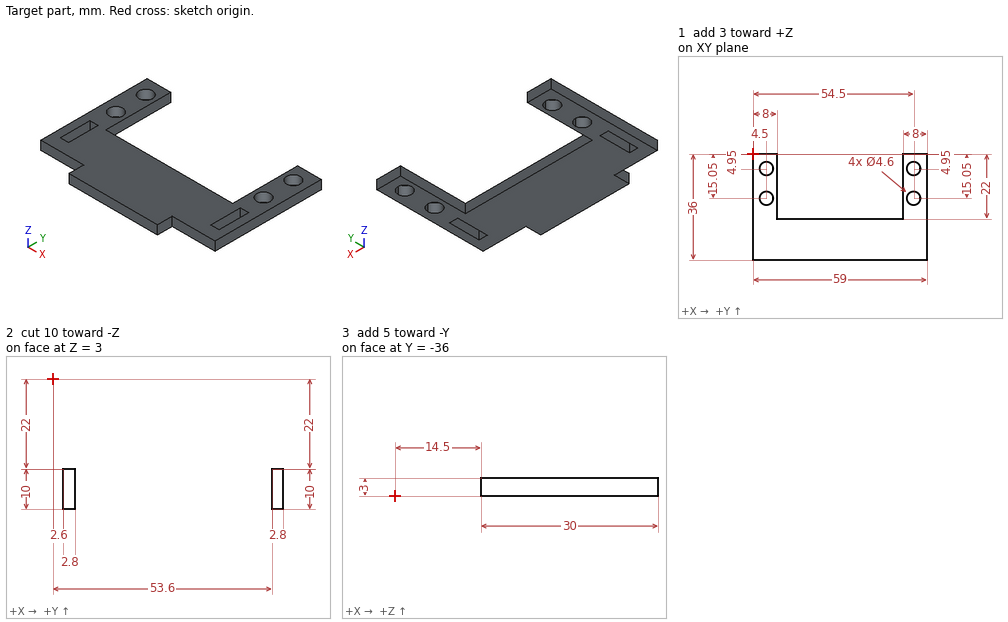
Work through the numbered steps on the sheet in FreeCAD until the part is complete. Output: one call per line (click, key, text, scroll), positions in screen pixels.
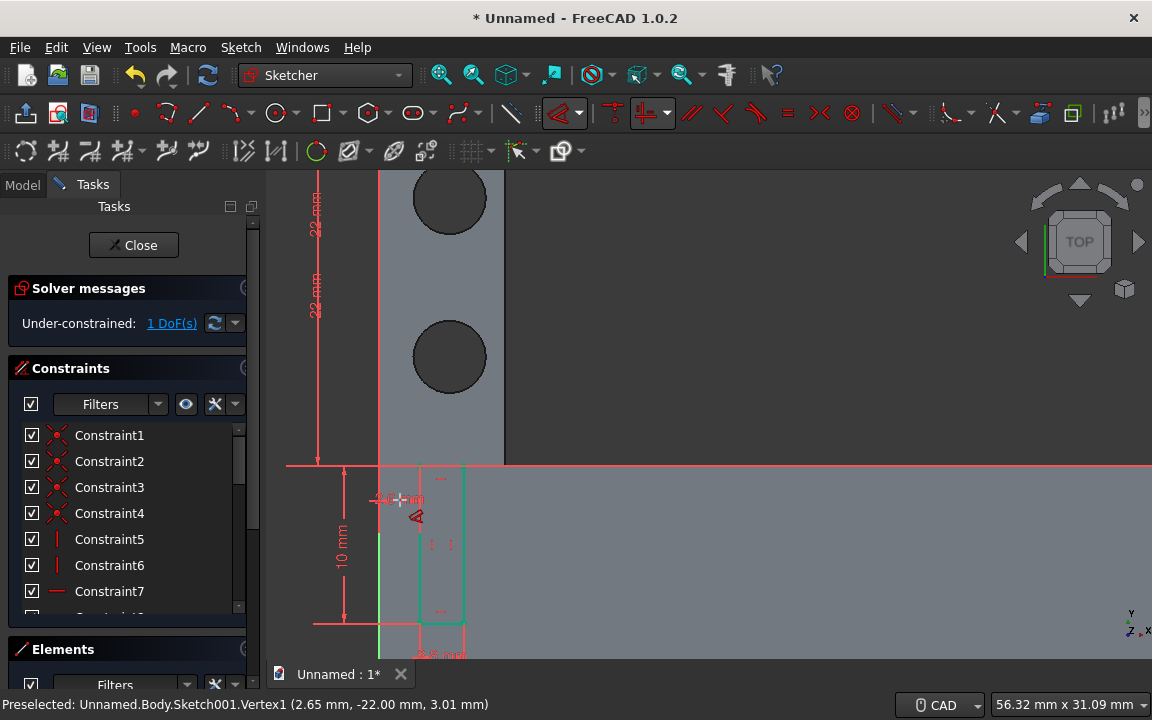
scroll(419, 466, down, 3)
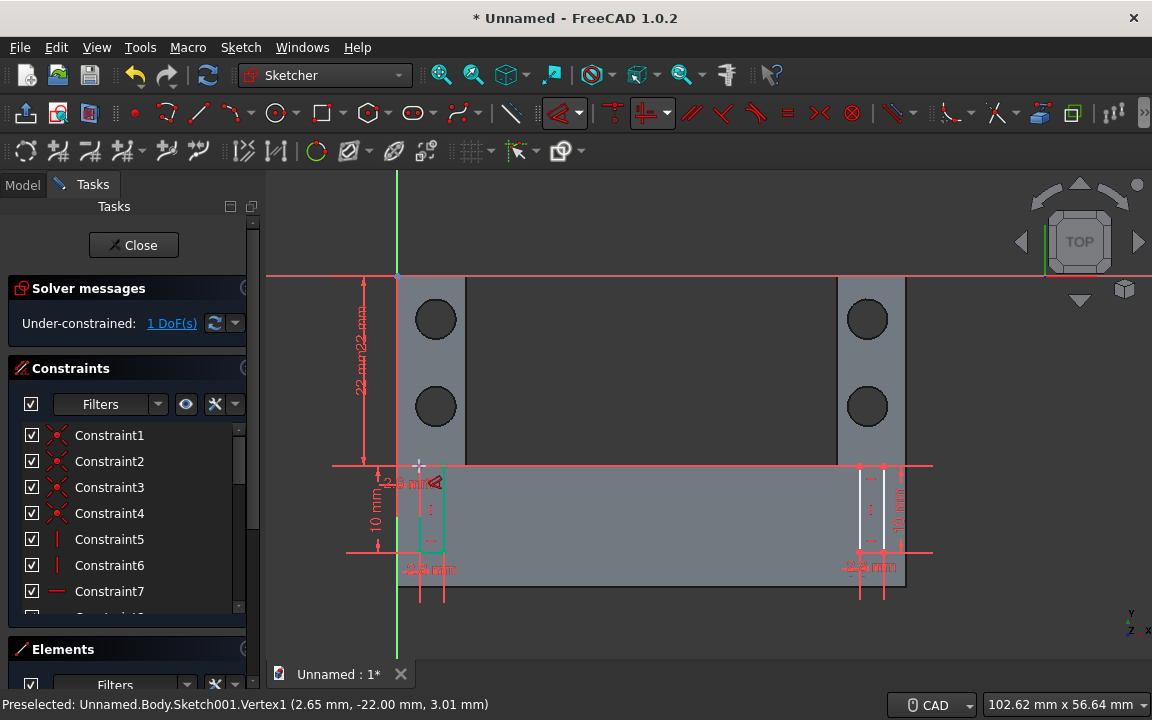
click(860, 466)
click(628, 242)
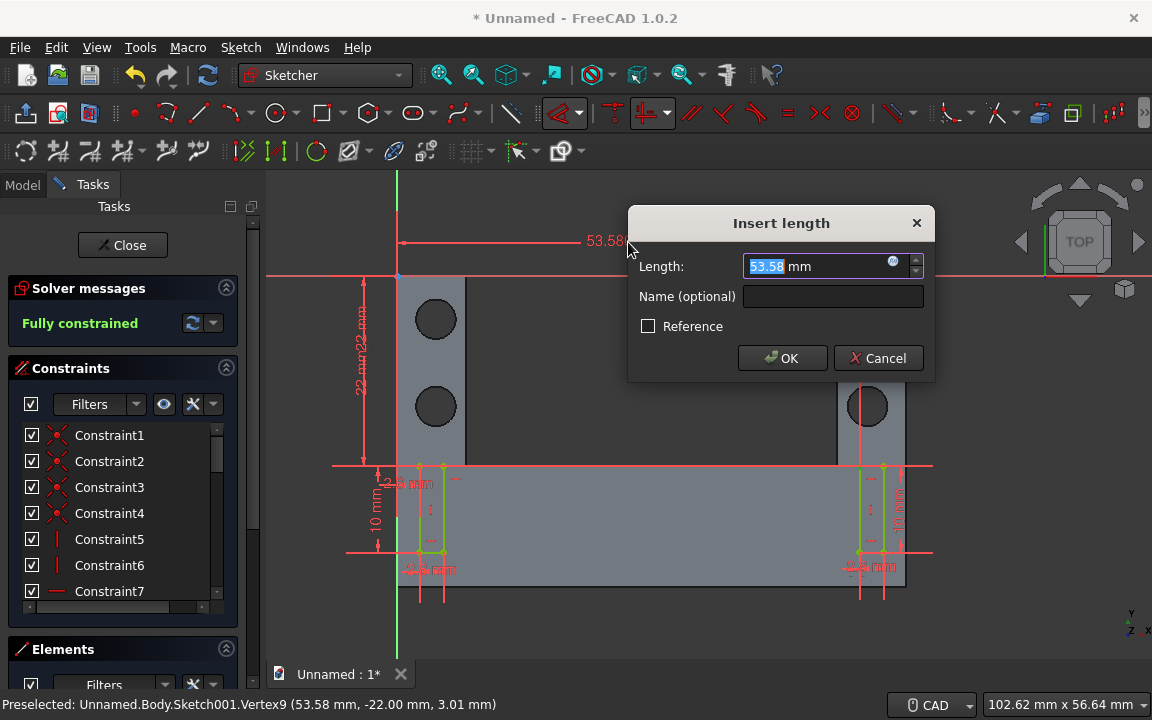
text(53.6)
key(Return)
key(Escape)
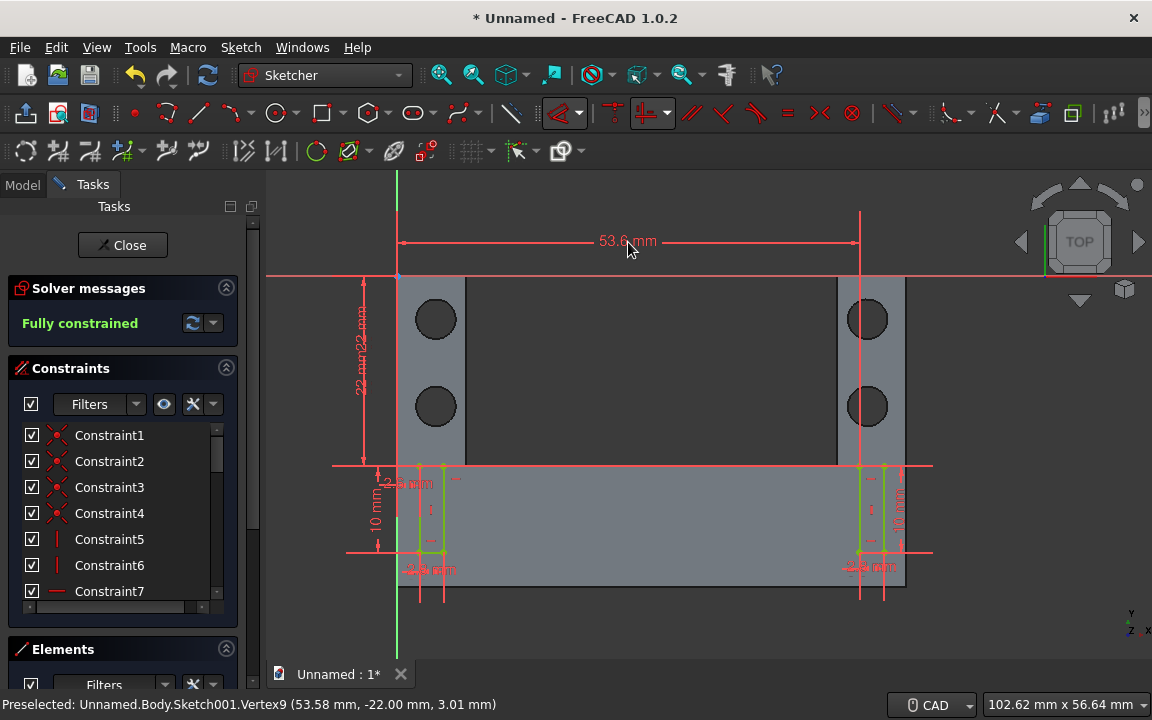
click(123, 245)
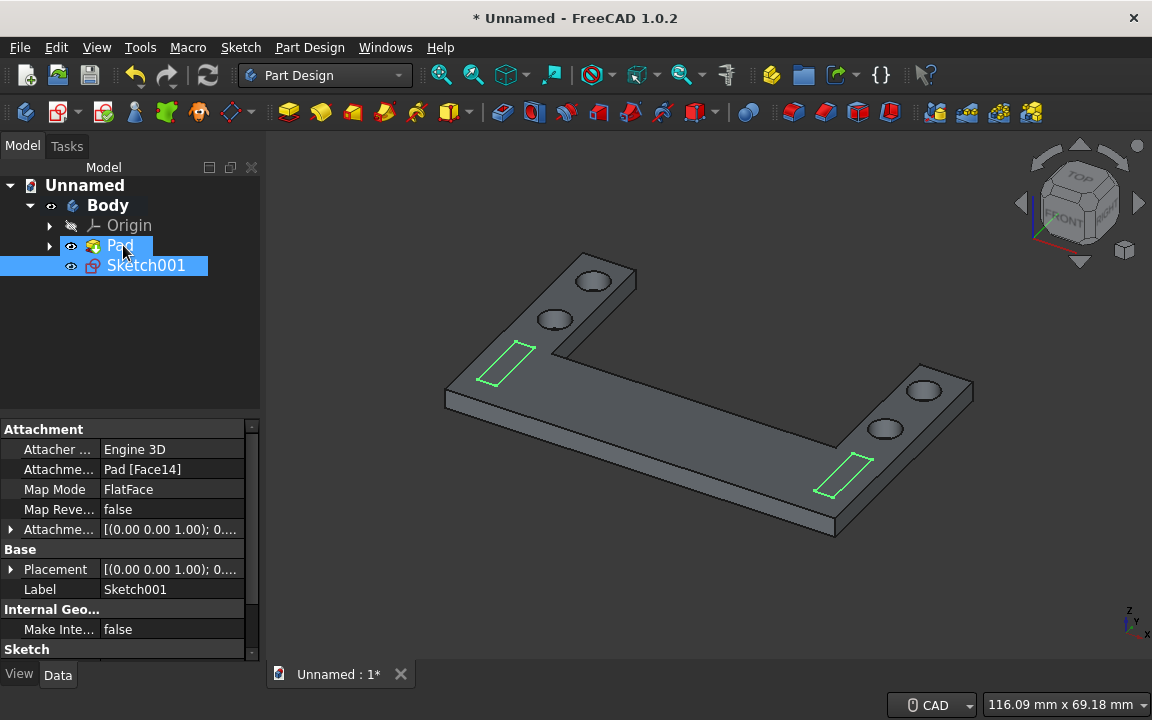
click(504, 112)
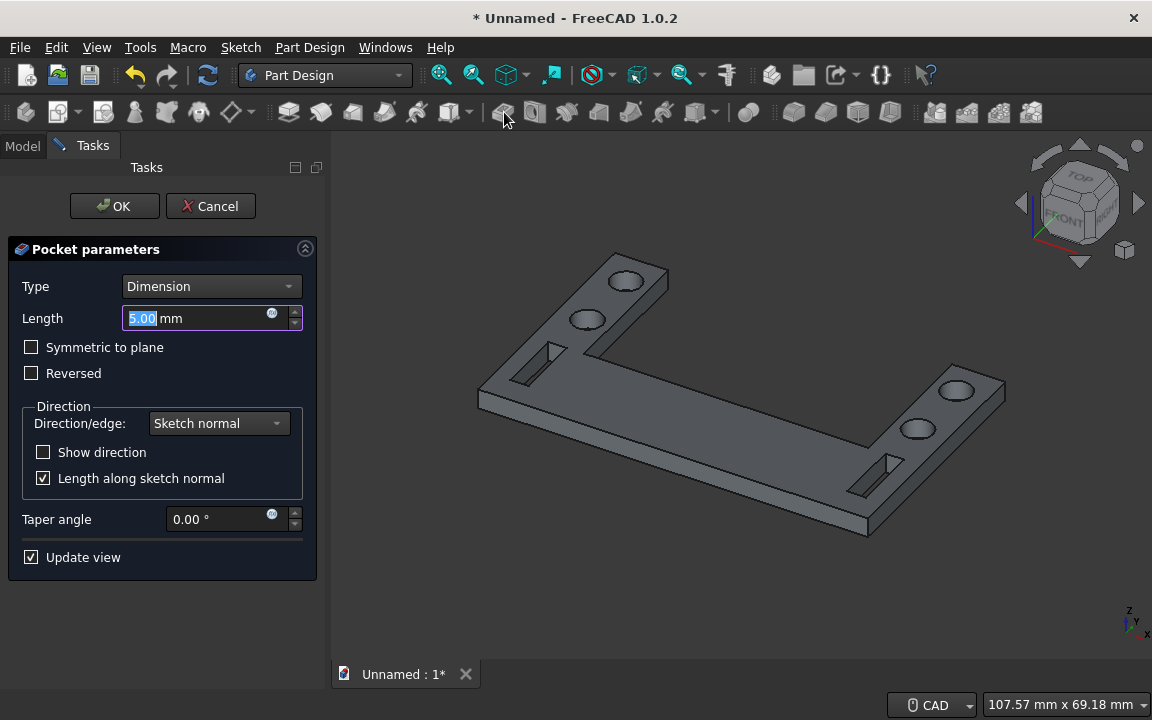
text(10)
key(Tab)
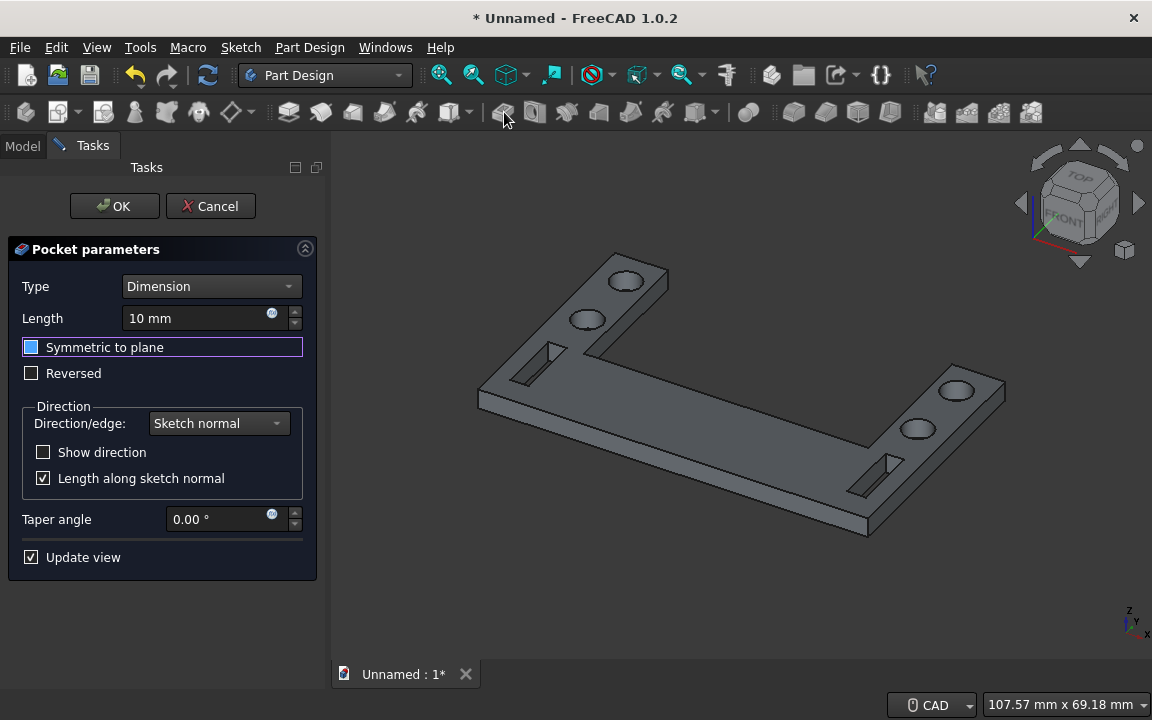
click(115, 206)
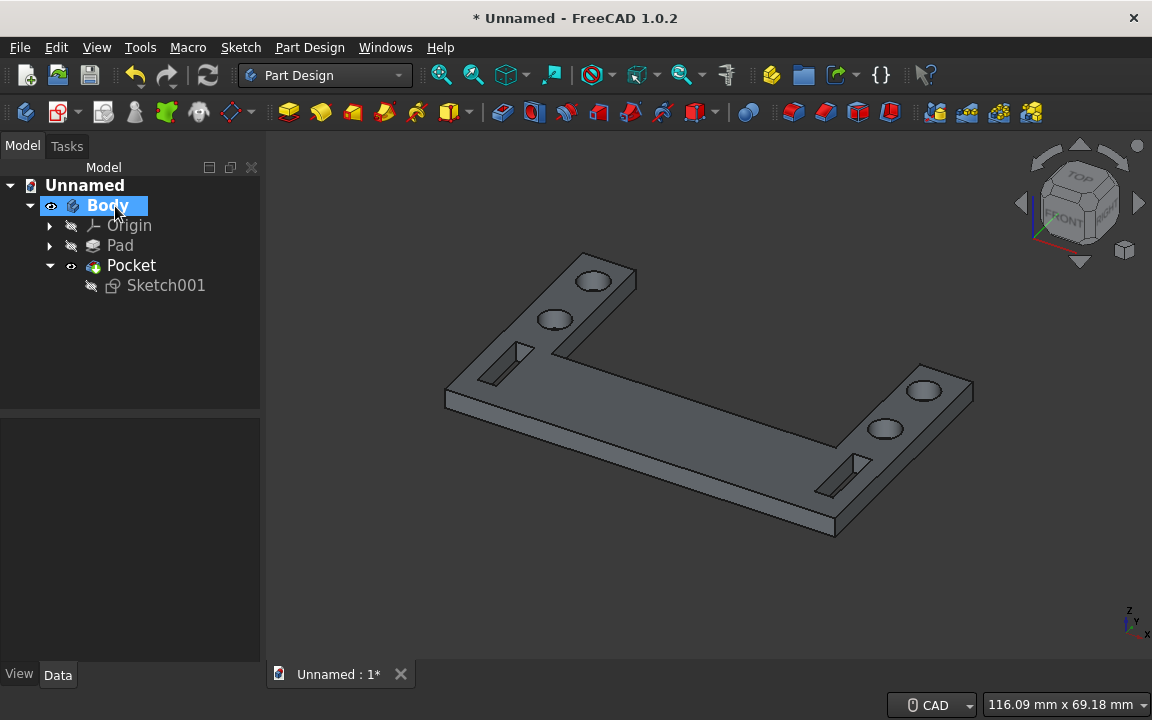
click(807, 518)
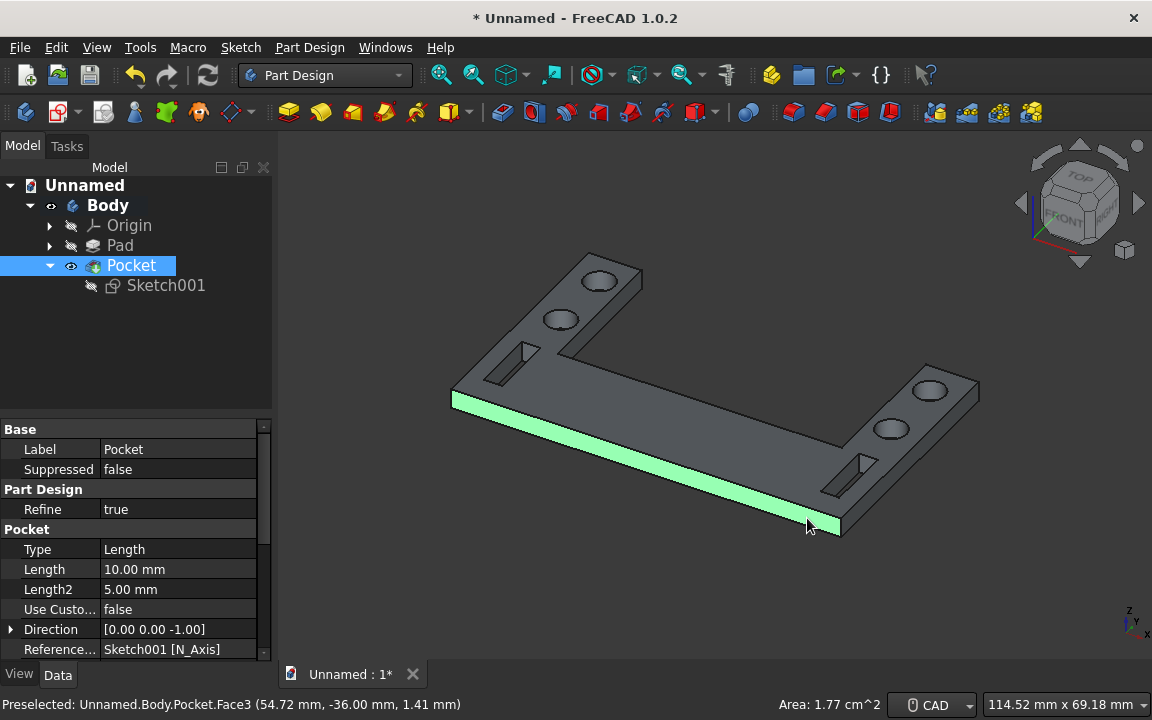
click(58, 112)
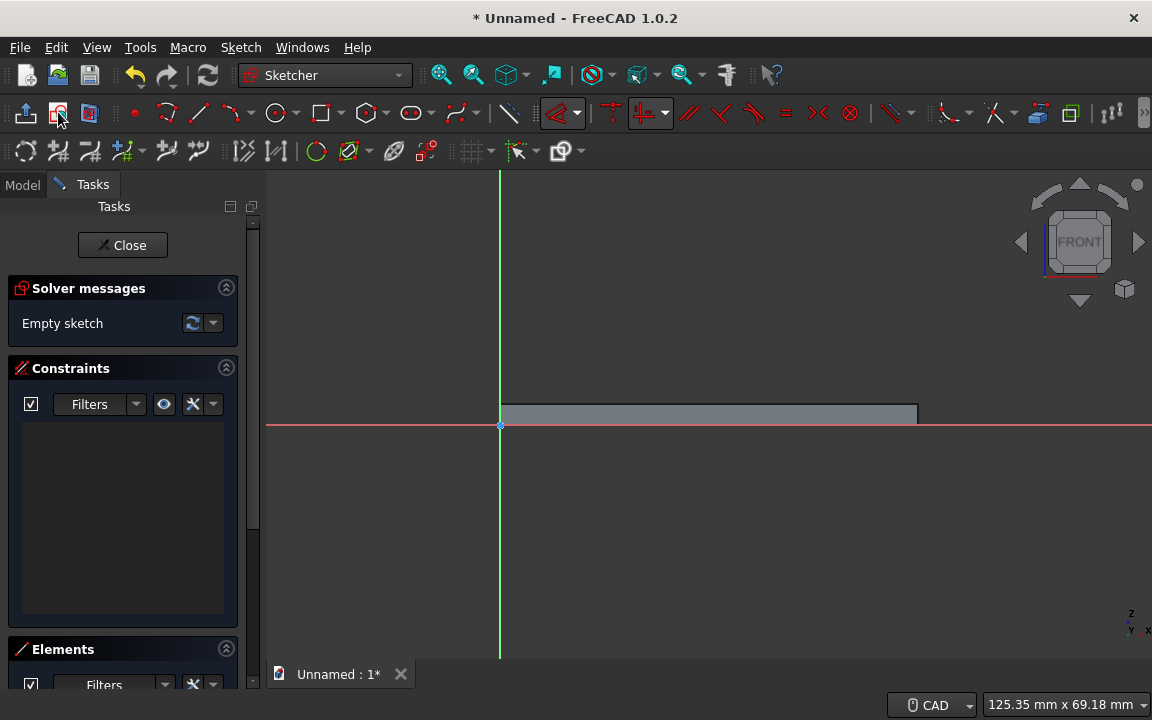
scroll(693, 414, up, 2)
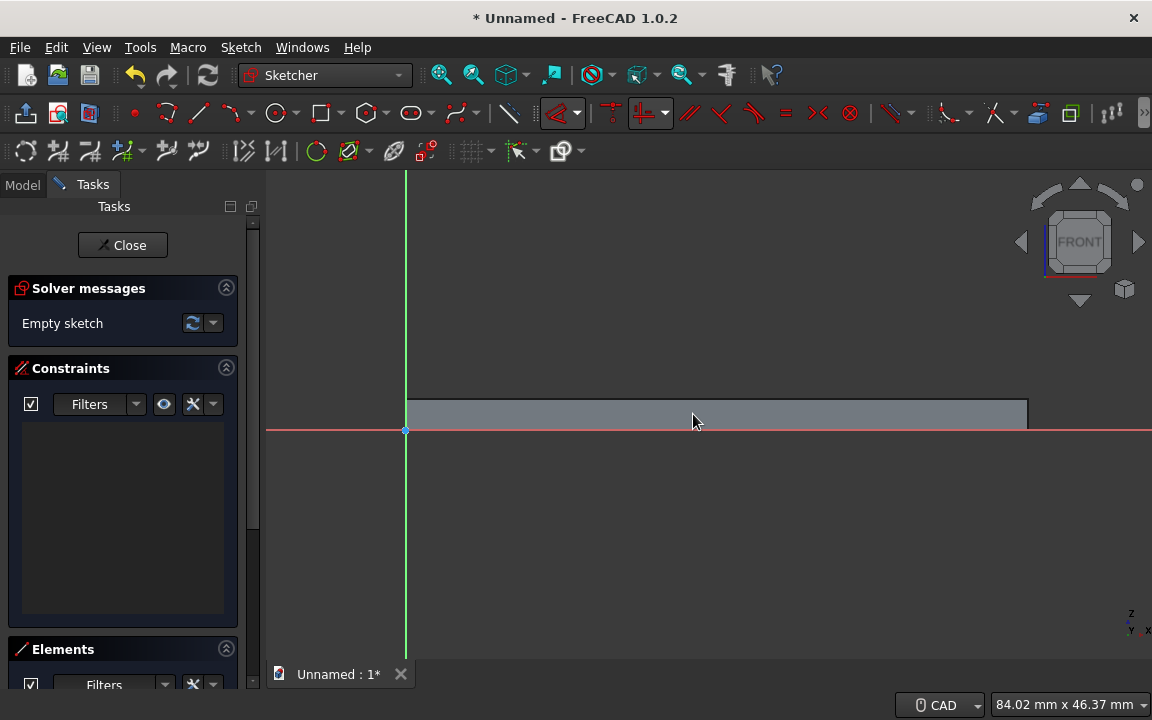
key(g)
key(r)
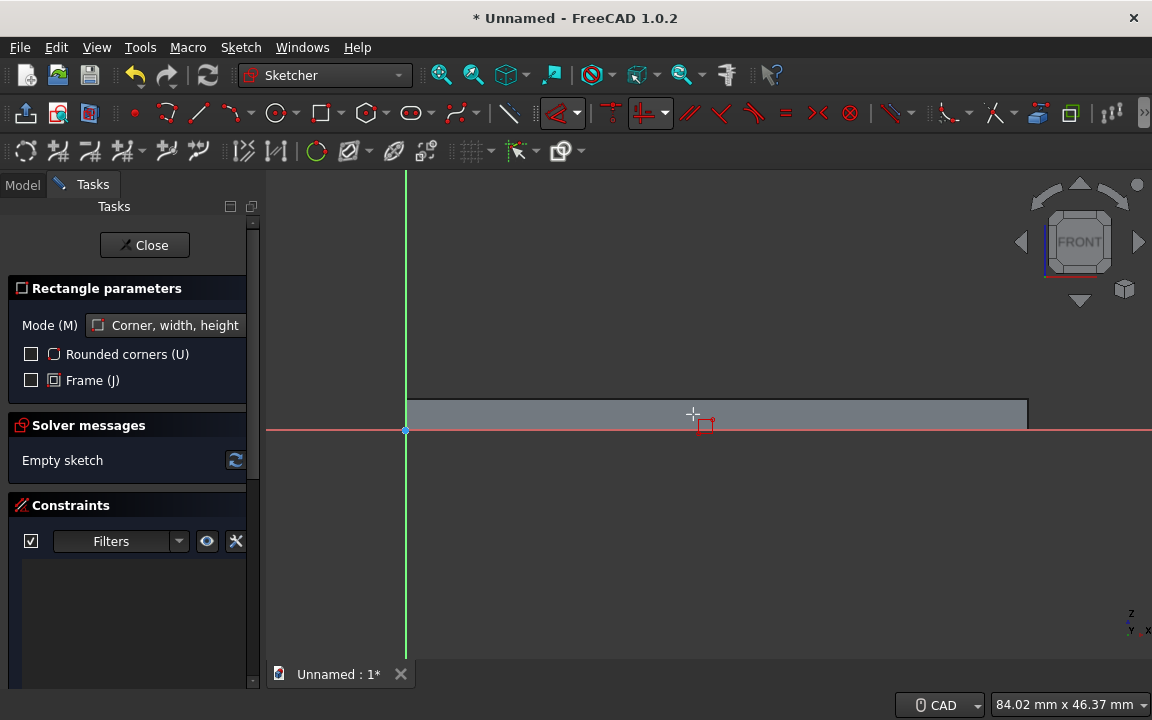
click(558, 399)
click(875, 430)
key(Escape)